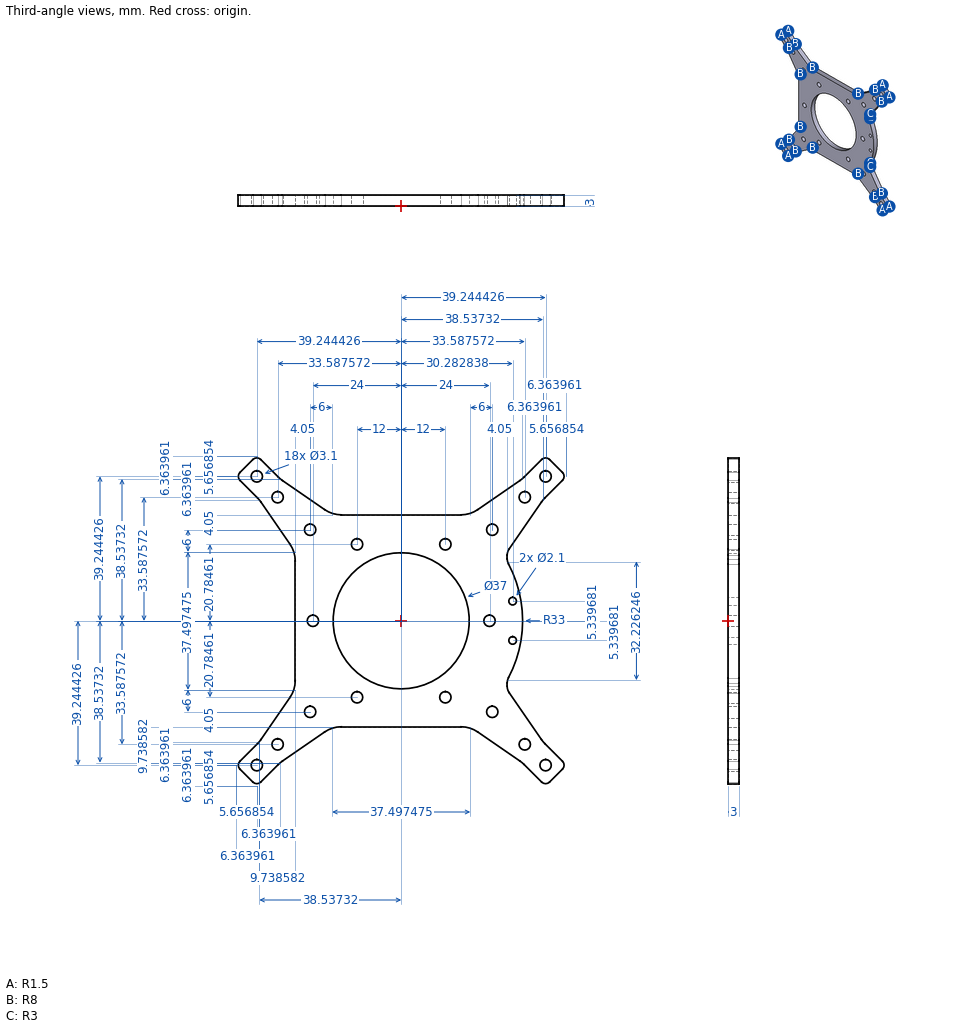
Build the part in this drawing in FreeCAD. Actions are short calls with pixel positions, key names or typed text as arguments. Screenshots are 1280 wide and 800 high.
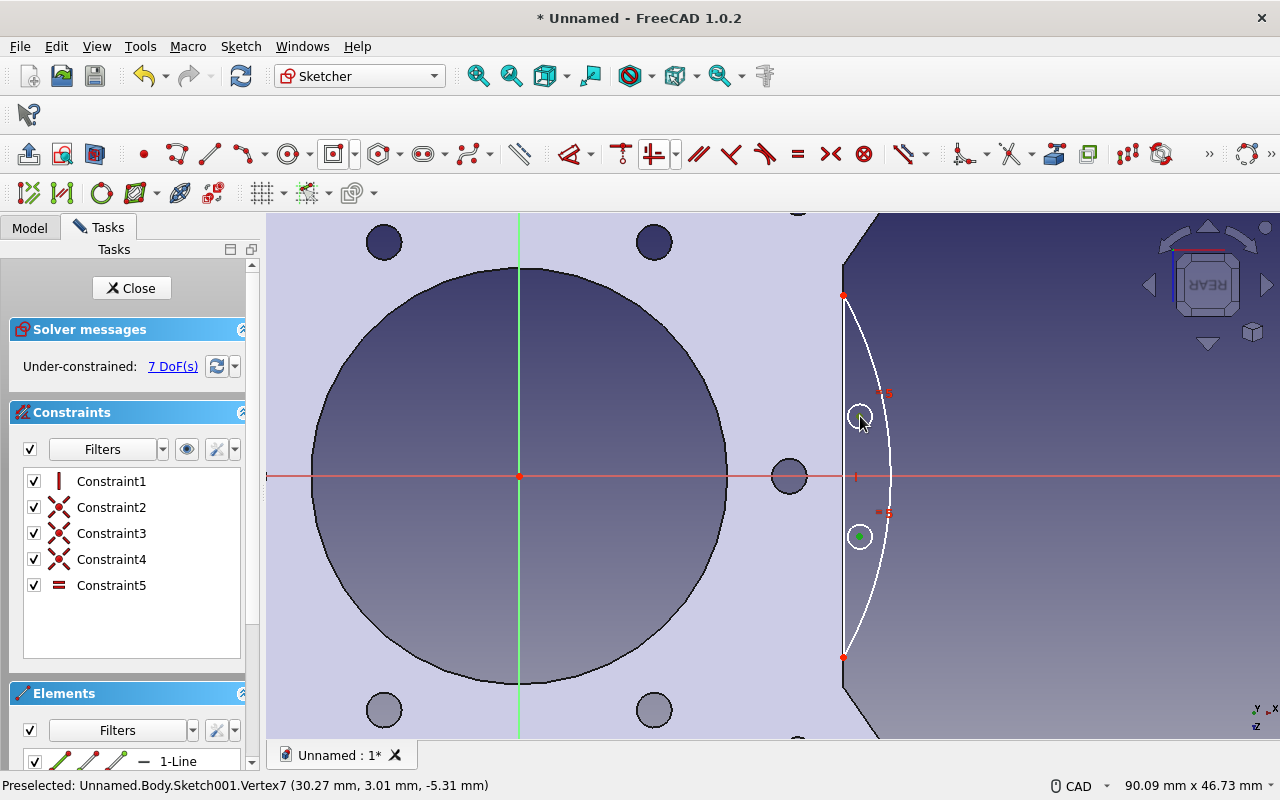
key(v)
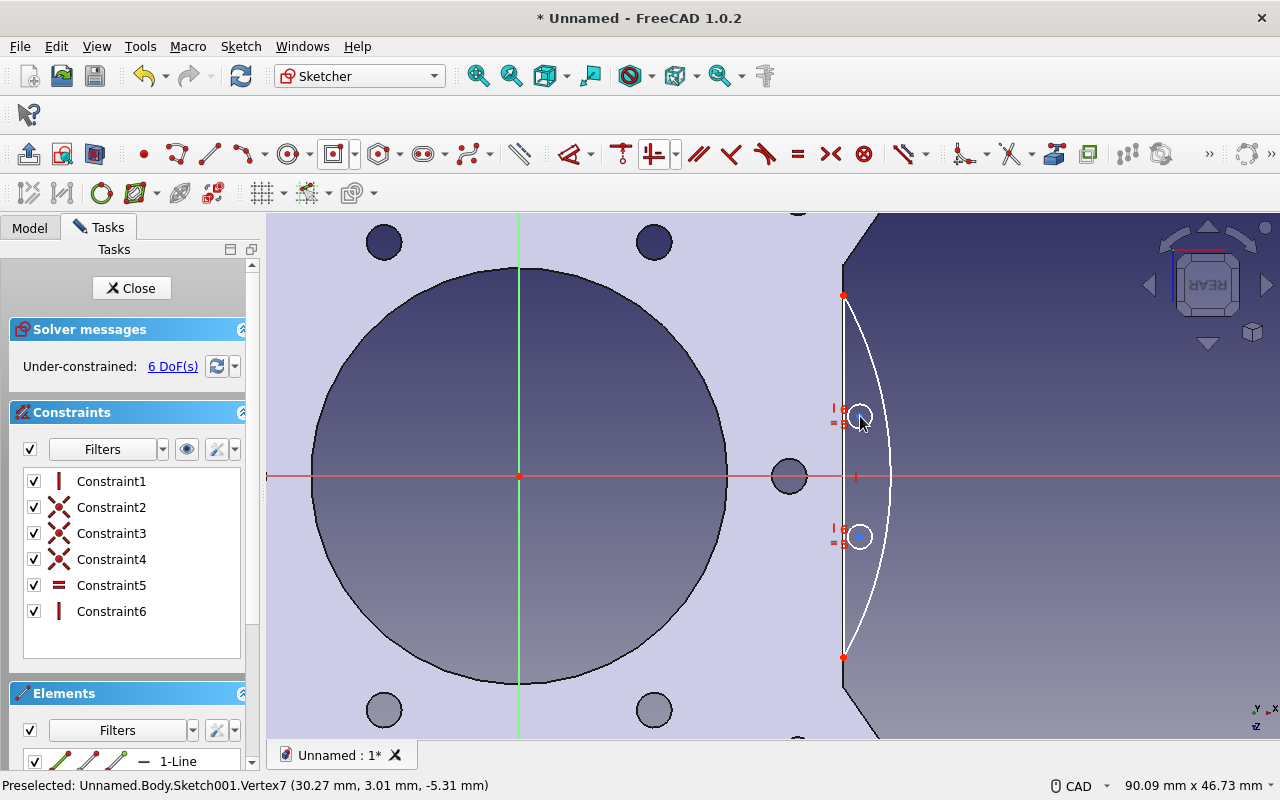
click(568, 154)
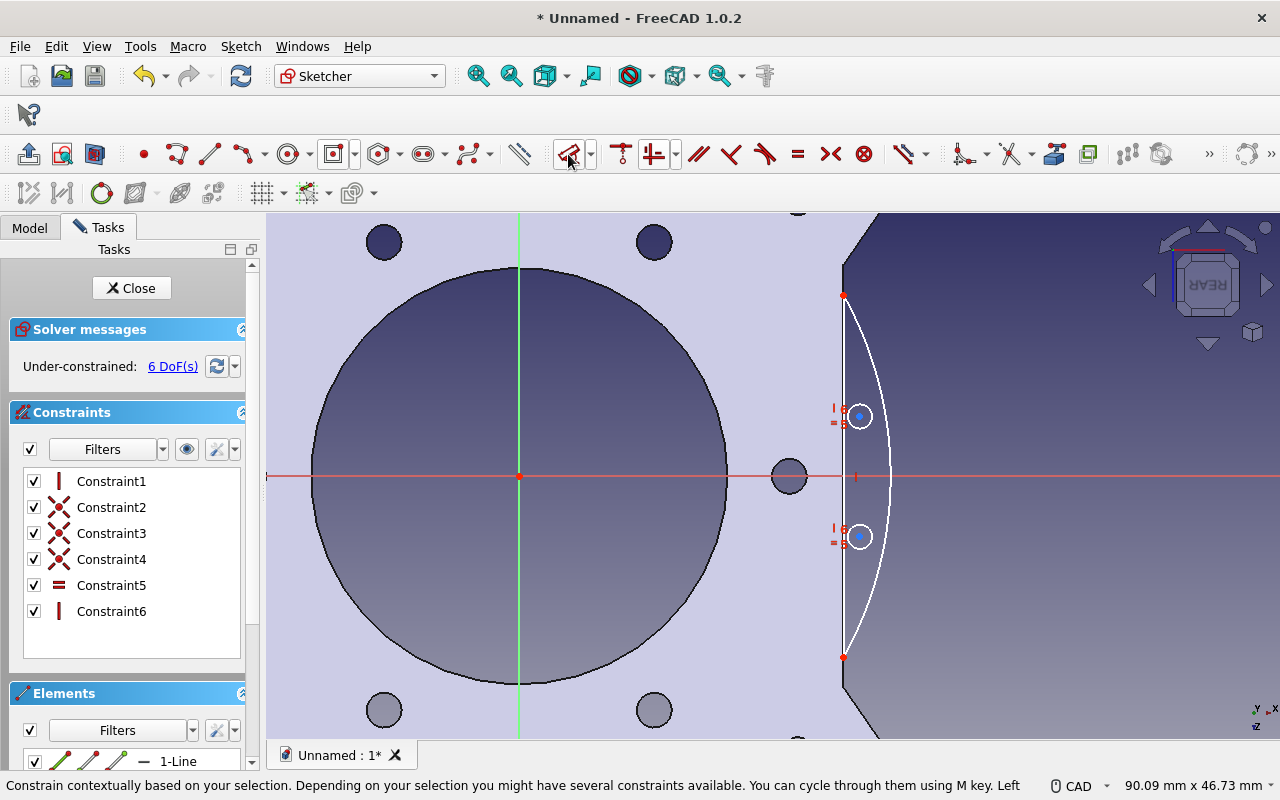
click(883, 551)
click(914, 557)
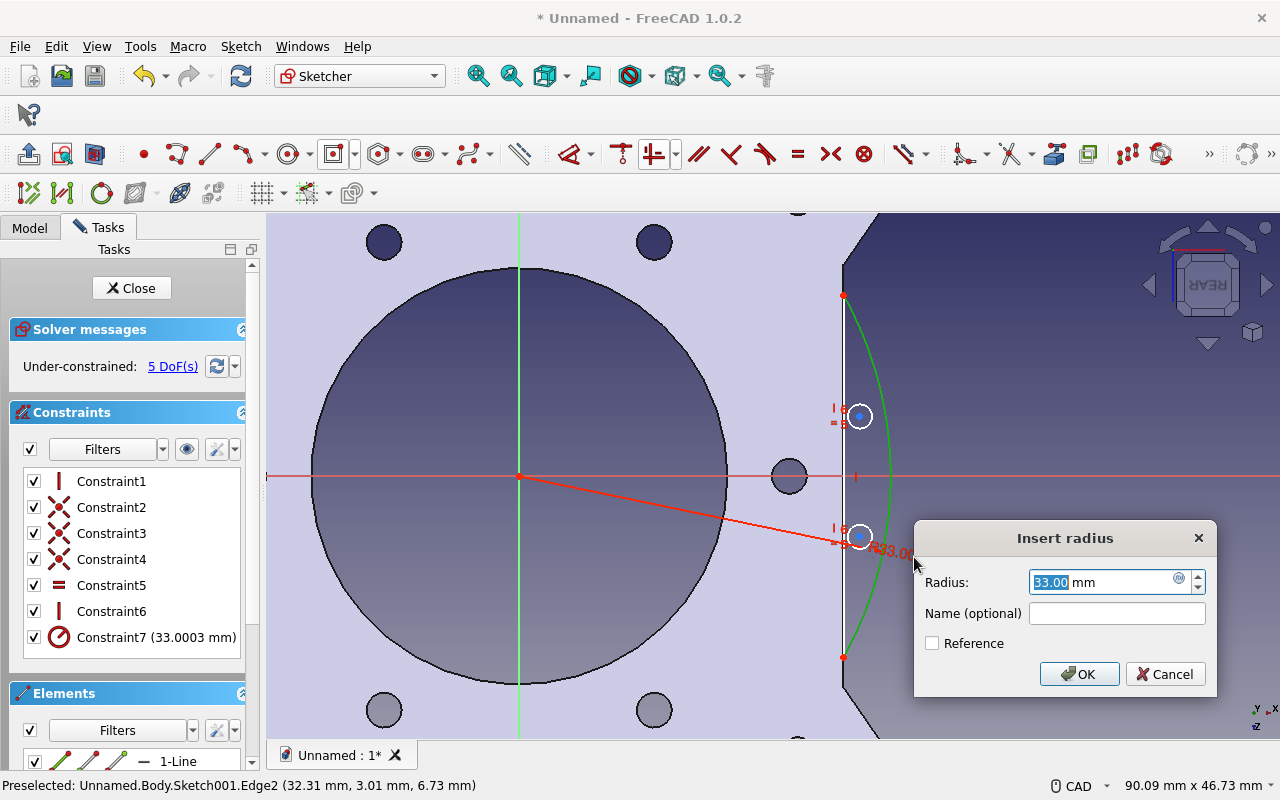
text(33)
key(Return)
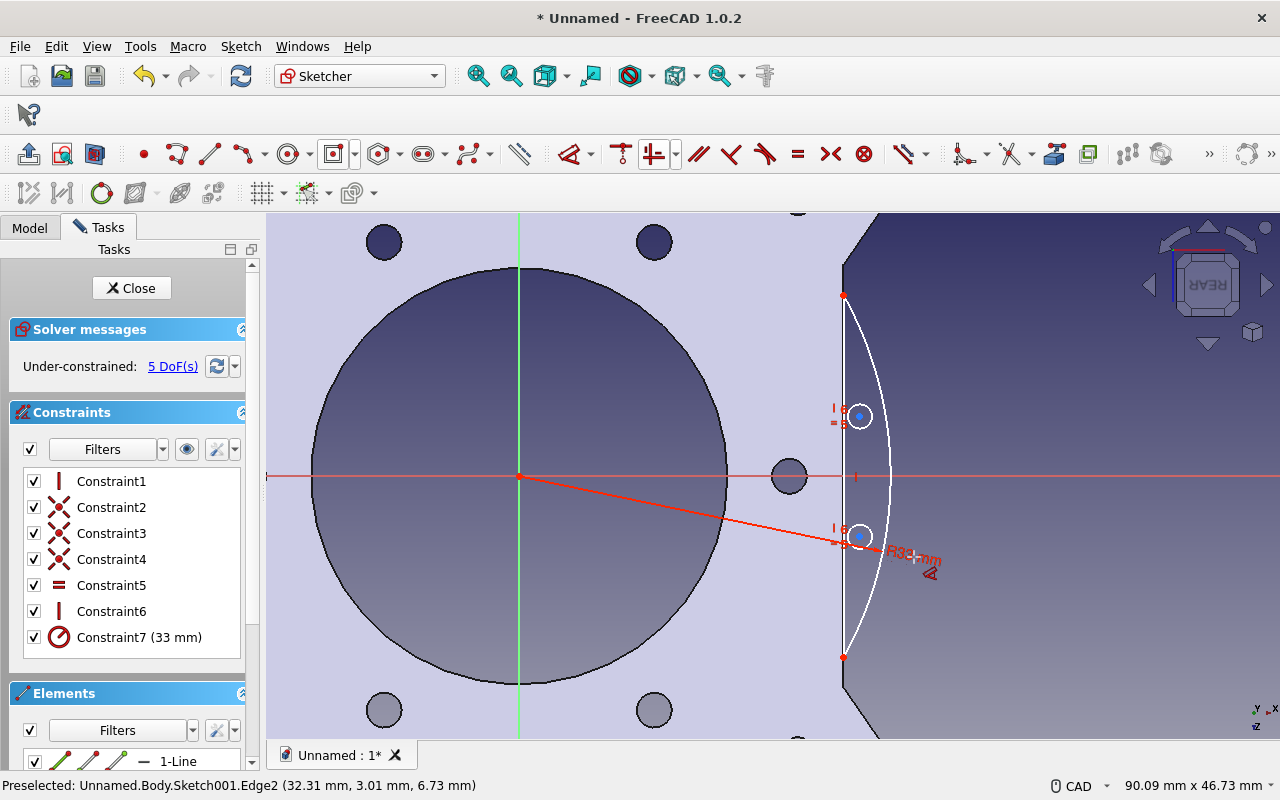
scroll(868, 528, up, 3)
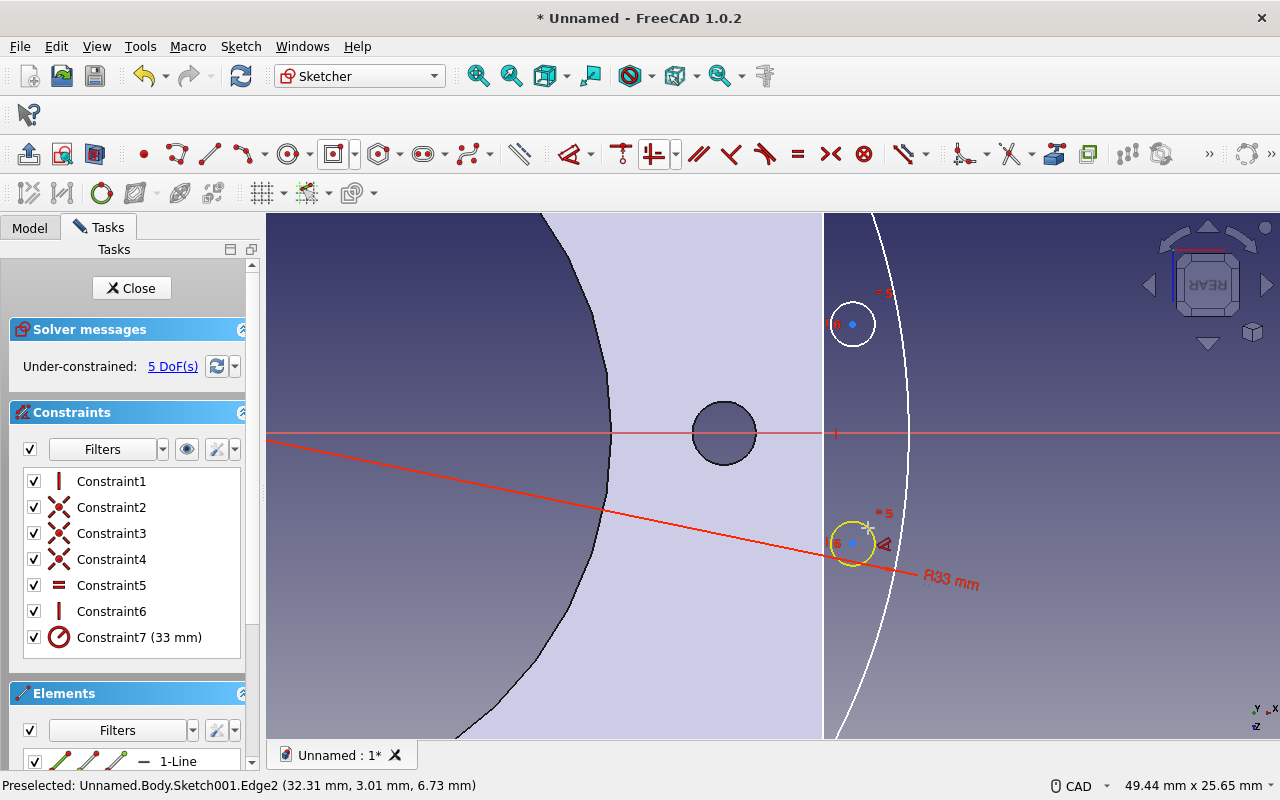
click(868, 528)
click(890, 505)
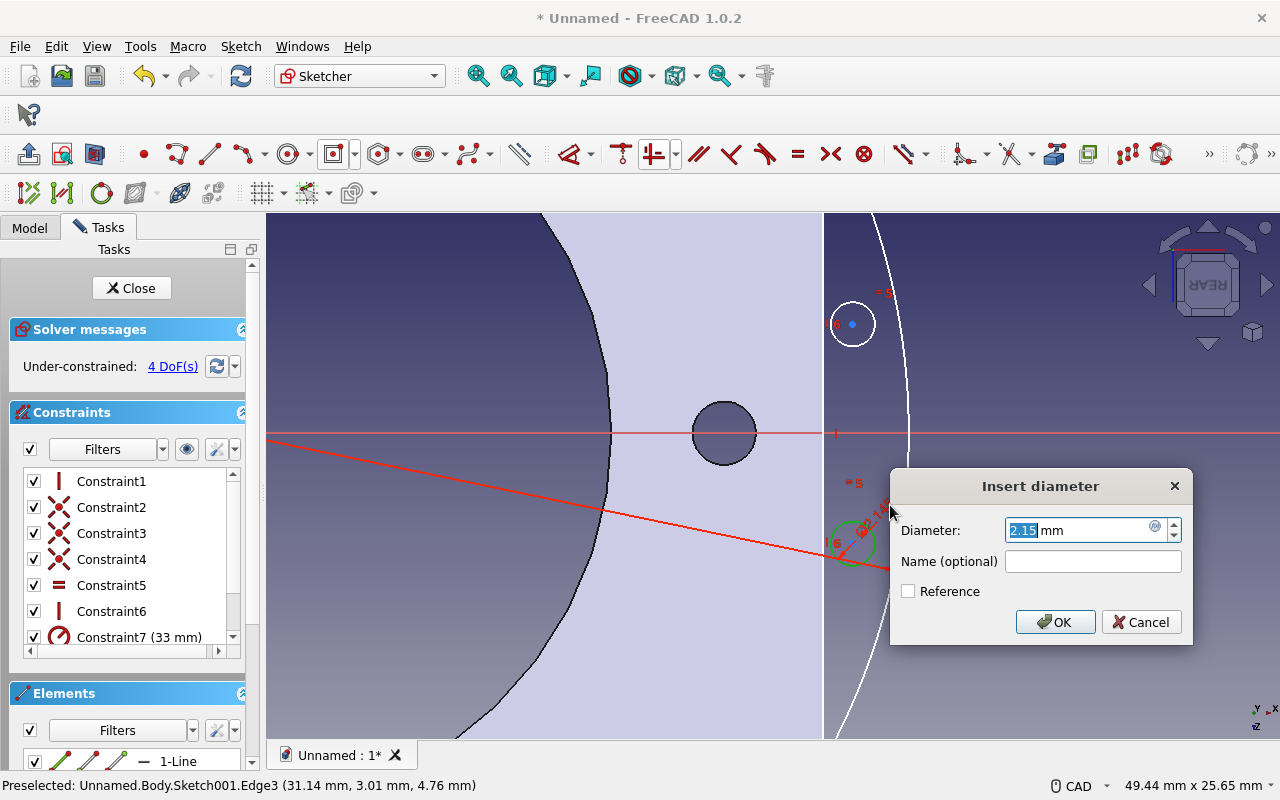
text(2.1)
key(Return)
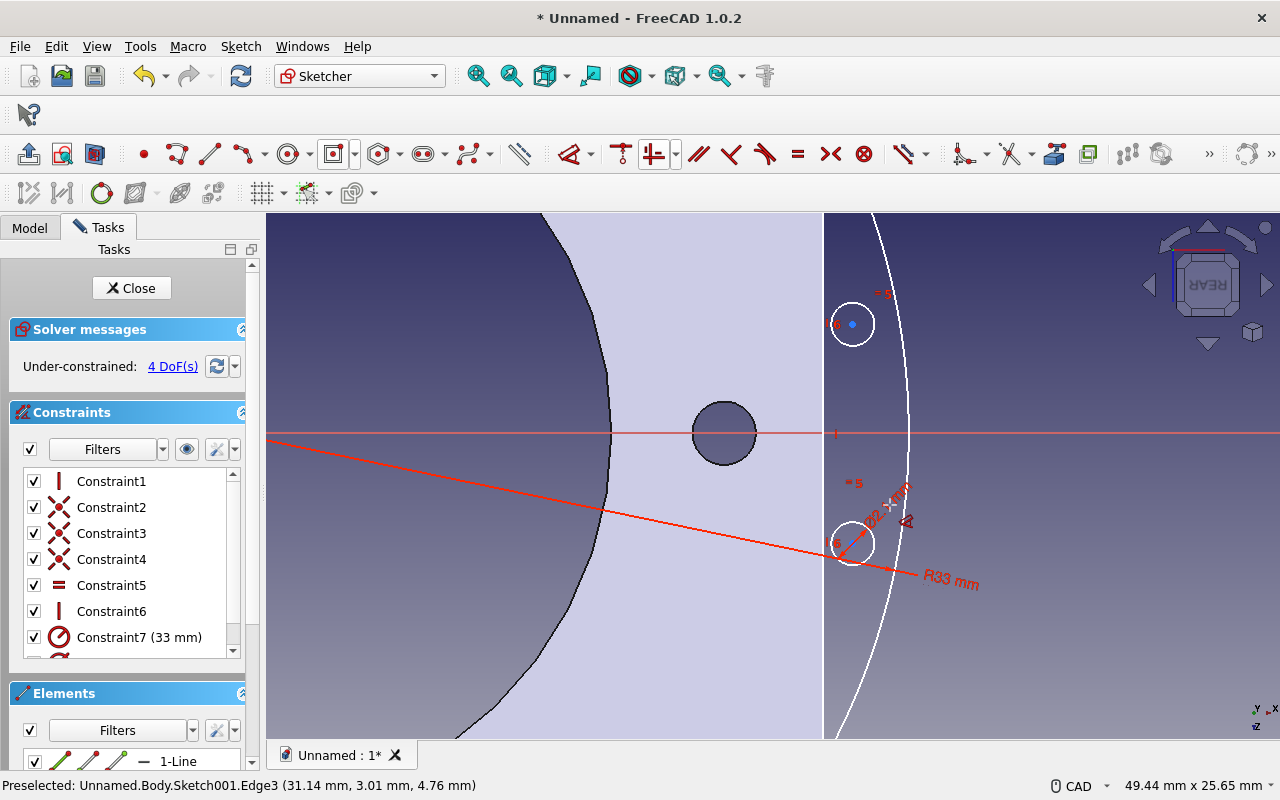
click(853, 544)
click(887, 463)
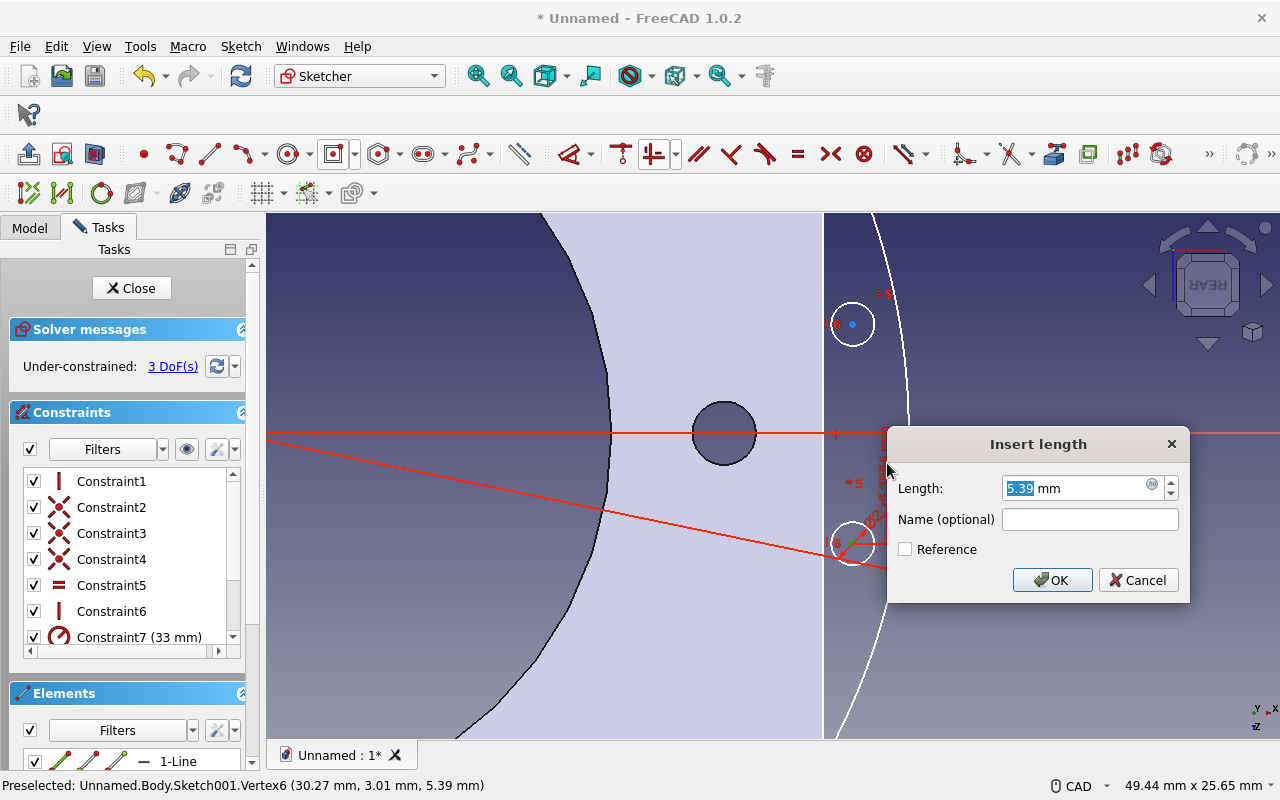
text(5.339681)
key(Return)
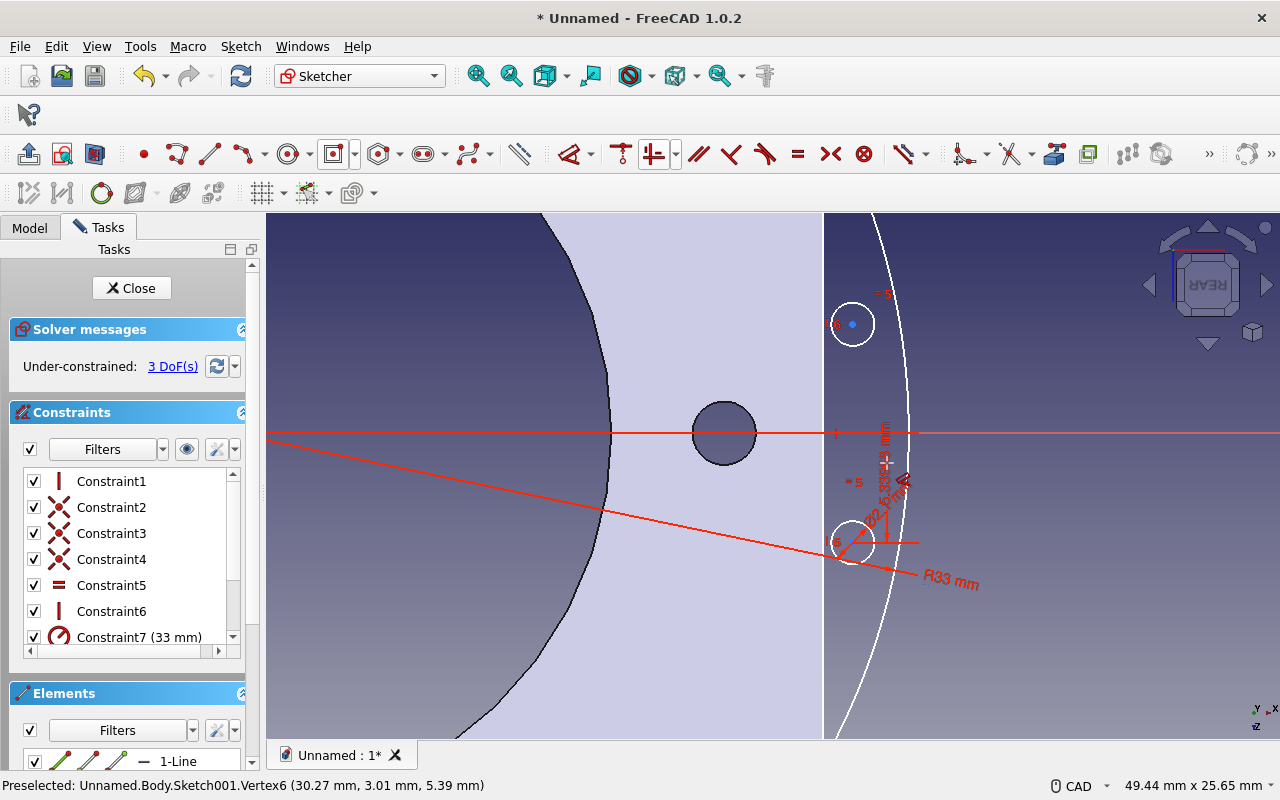
click(853, 324)
click(887, 379)